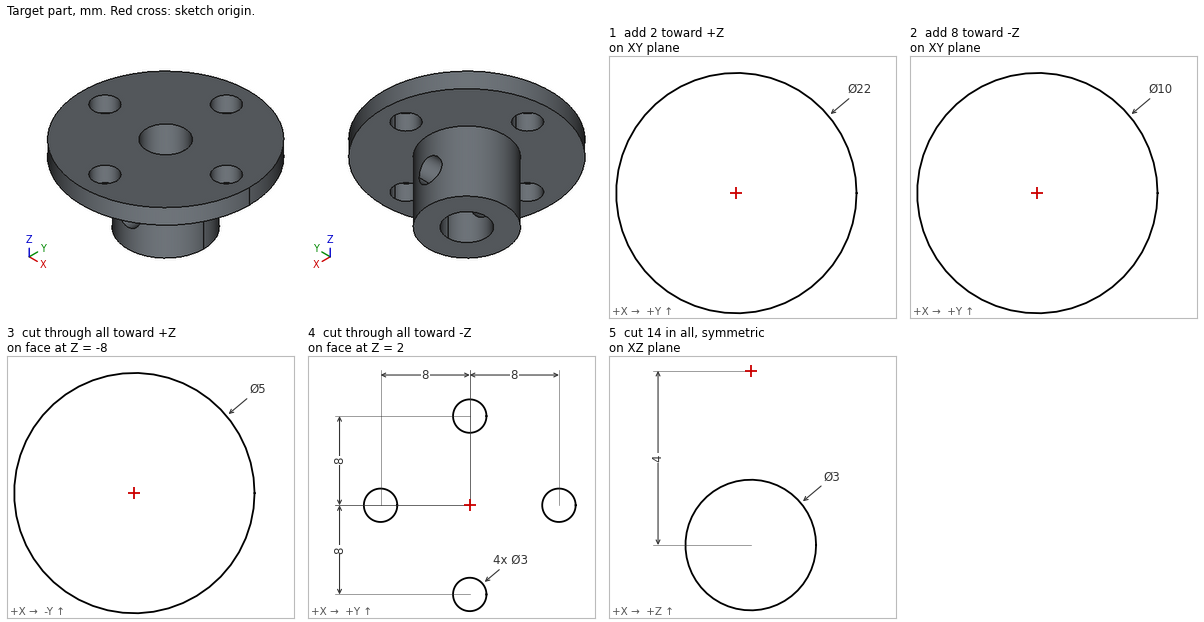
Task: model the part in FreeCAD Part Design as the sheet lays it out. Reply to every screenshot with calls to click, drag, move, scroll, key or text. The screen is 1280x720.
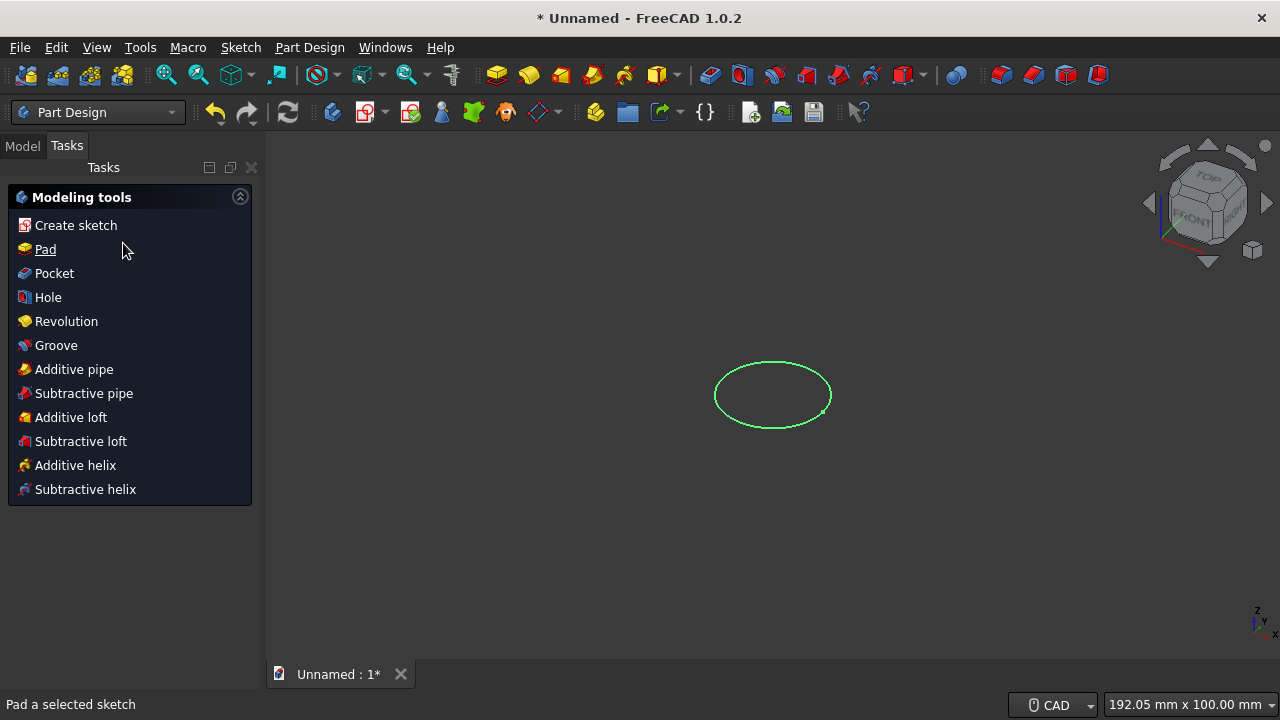
click(498, 76)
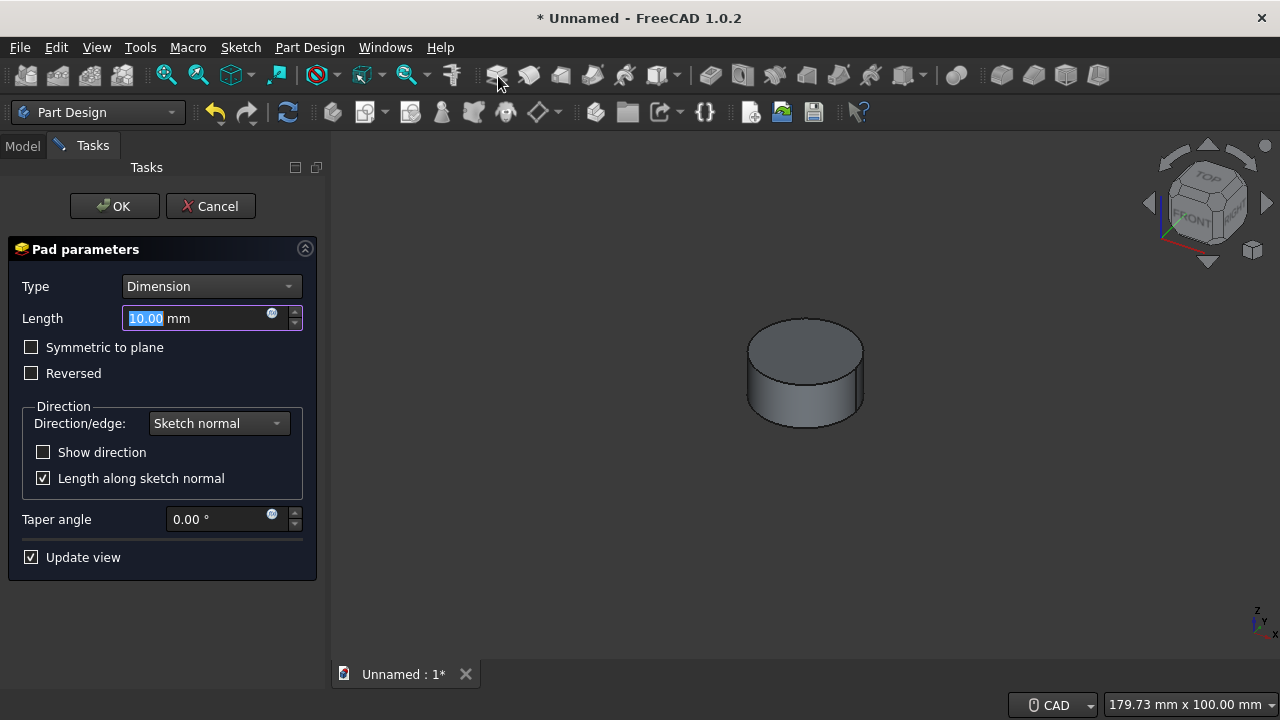
text(2)
key(Tab)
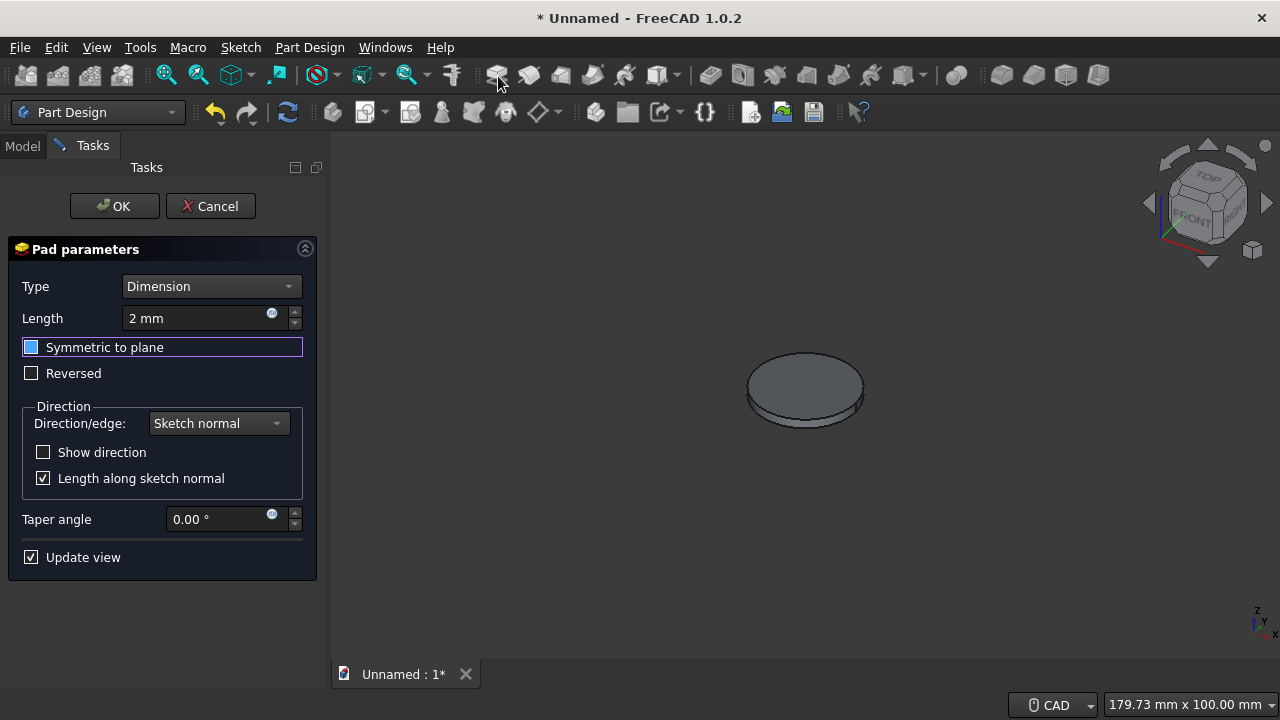
click(115, 206)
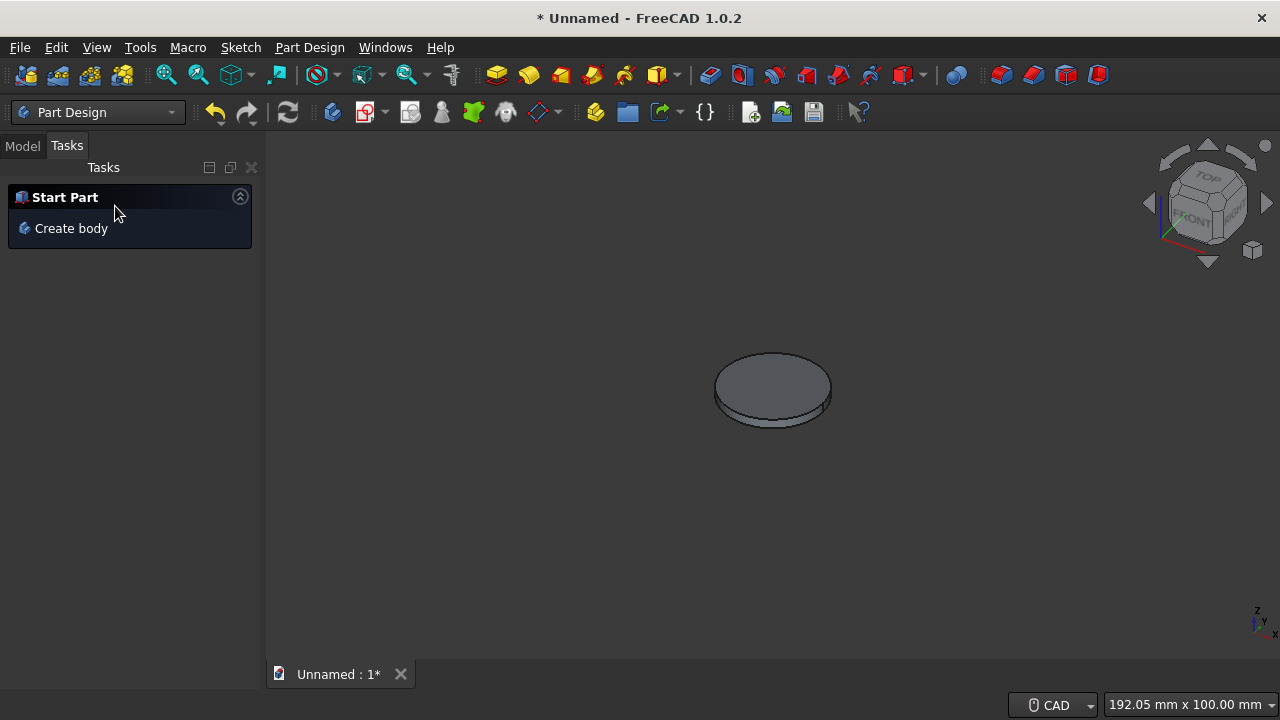
key(v)
key(f)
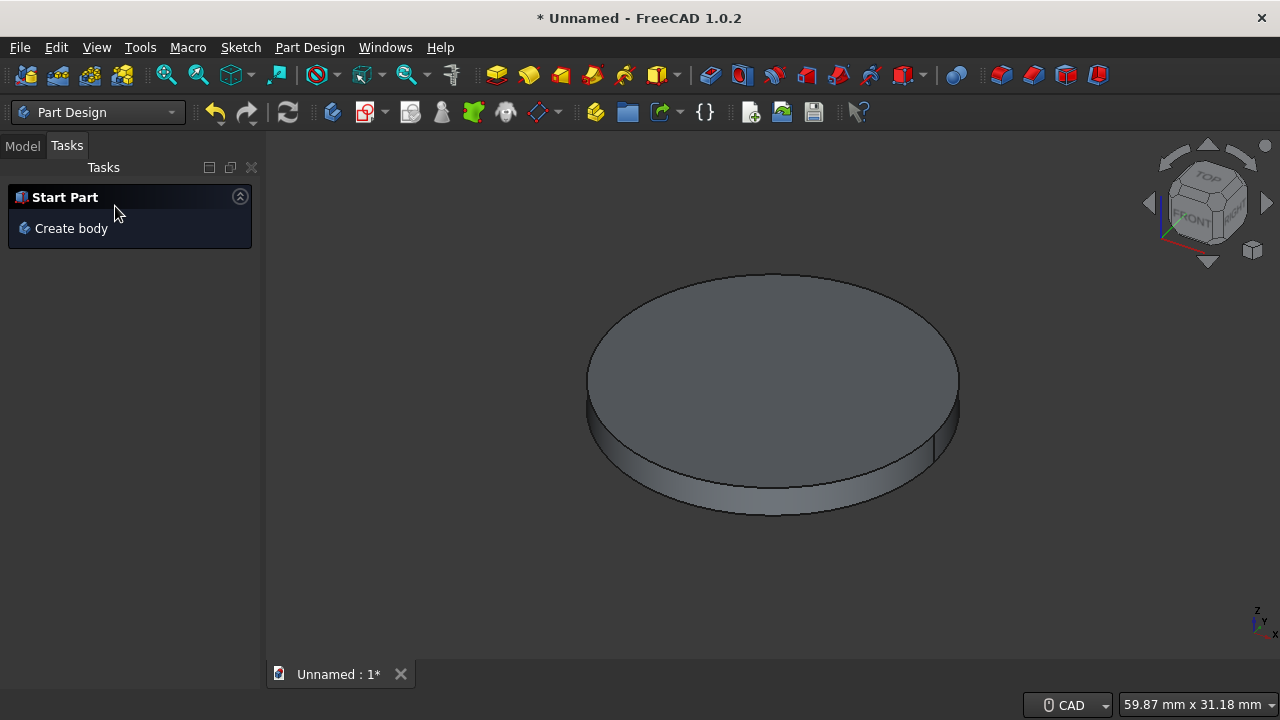
click(366, 112)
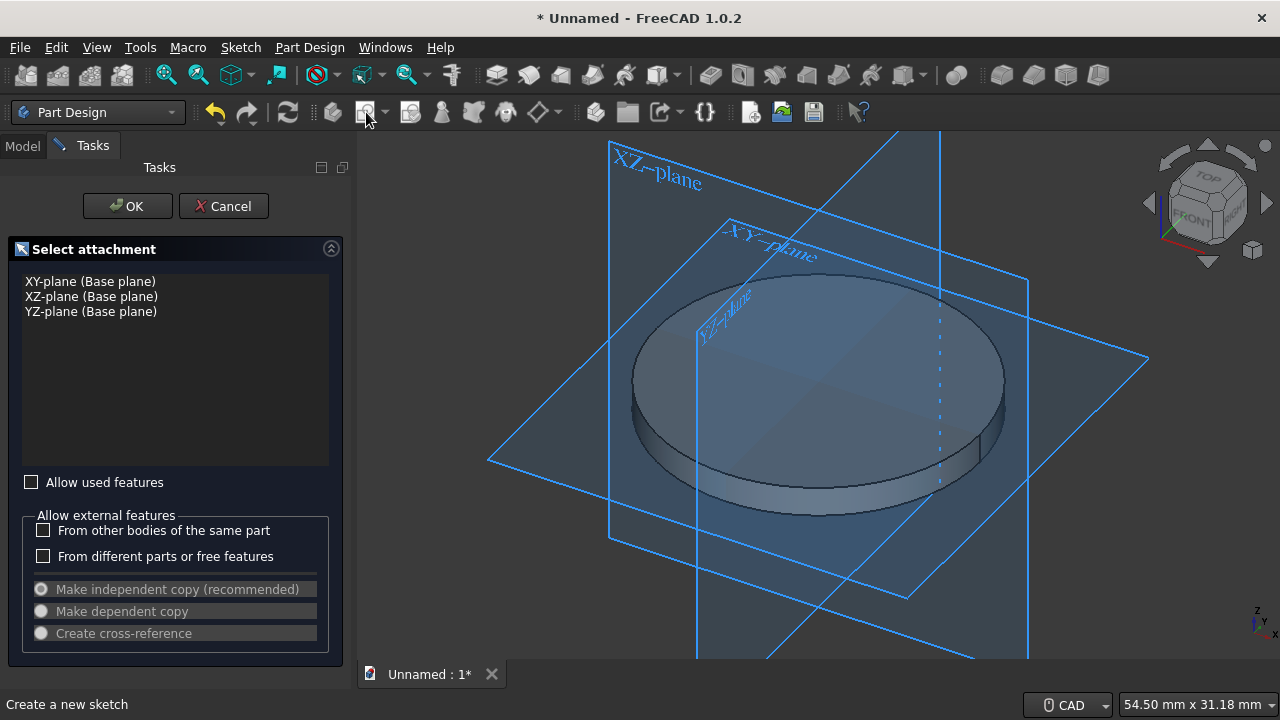
click(82, 282)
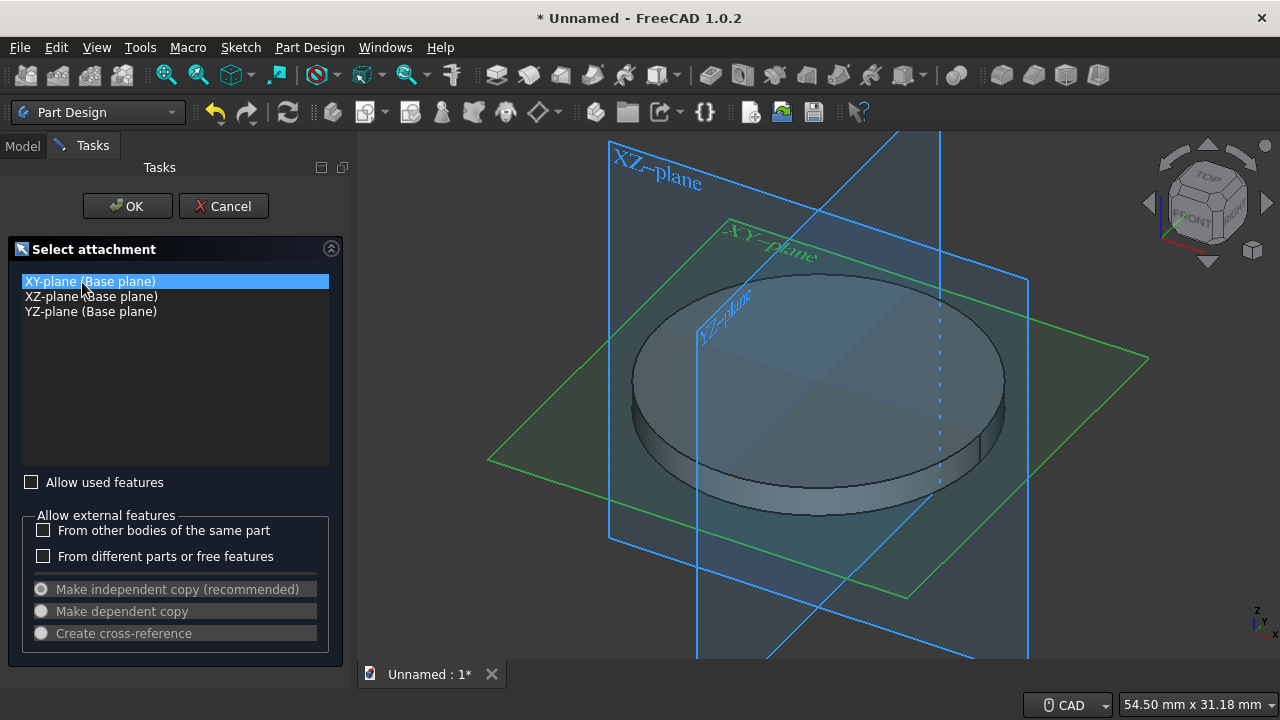
click(128, 206)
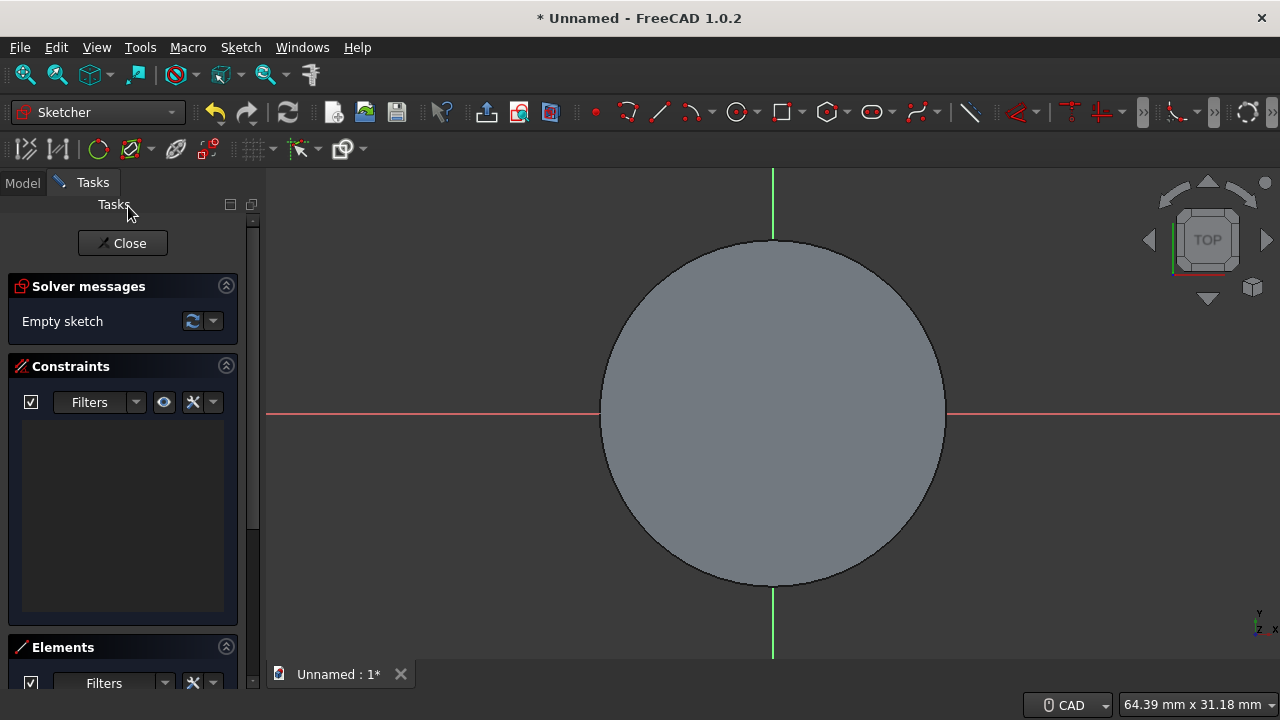
key(q)
key(s)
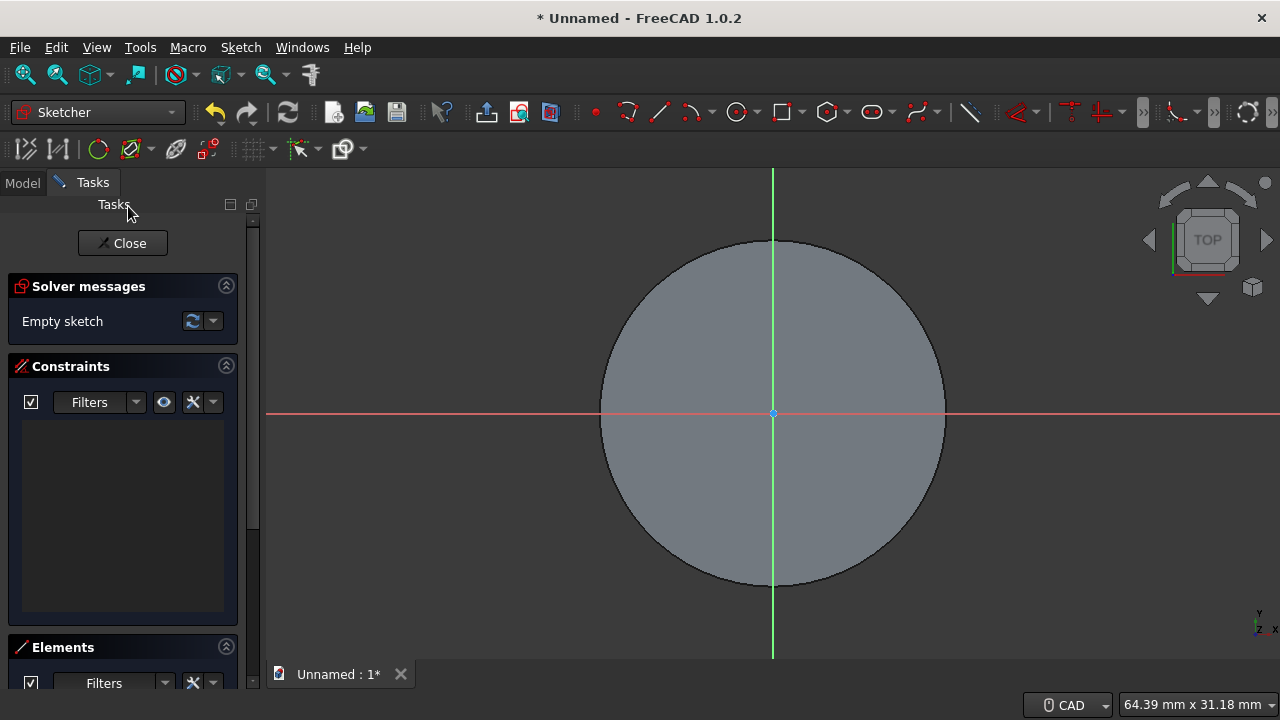
scroll(856, 414, up, 3)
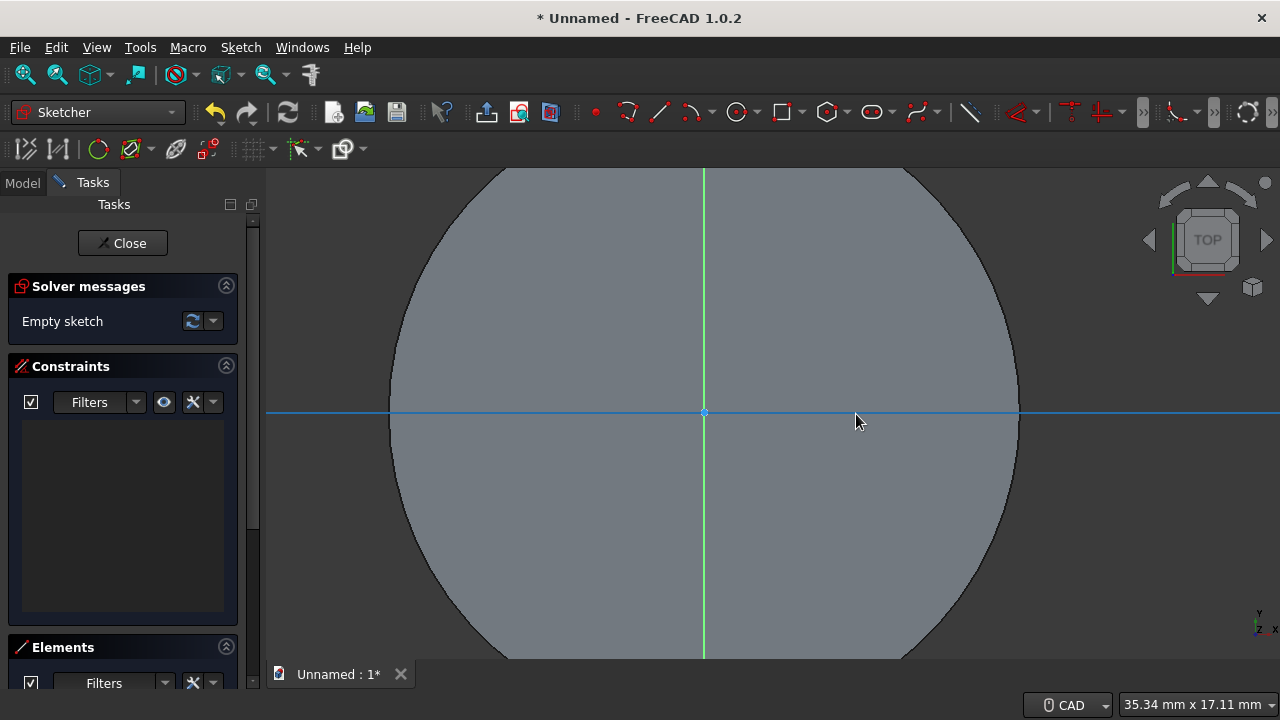
key(g)
key(c)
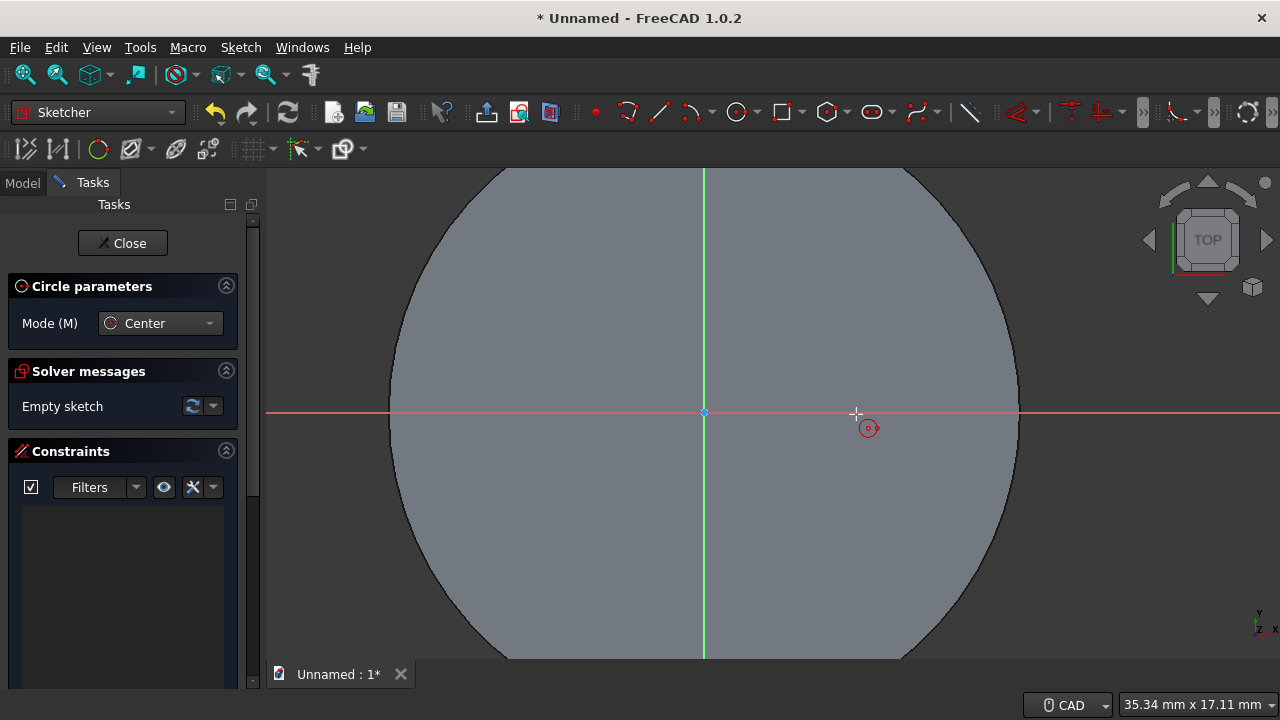
click(704, 413)
click(806, 311)
key(Escape)